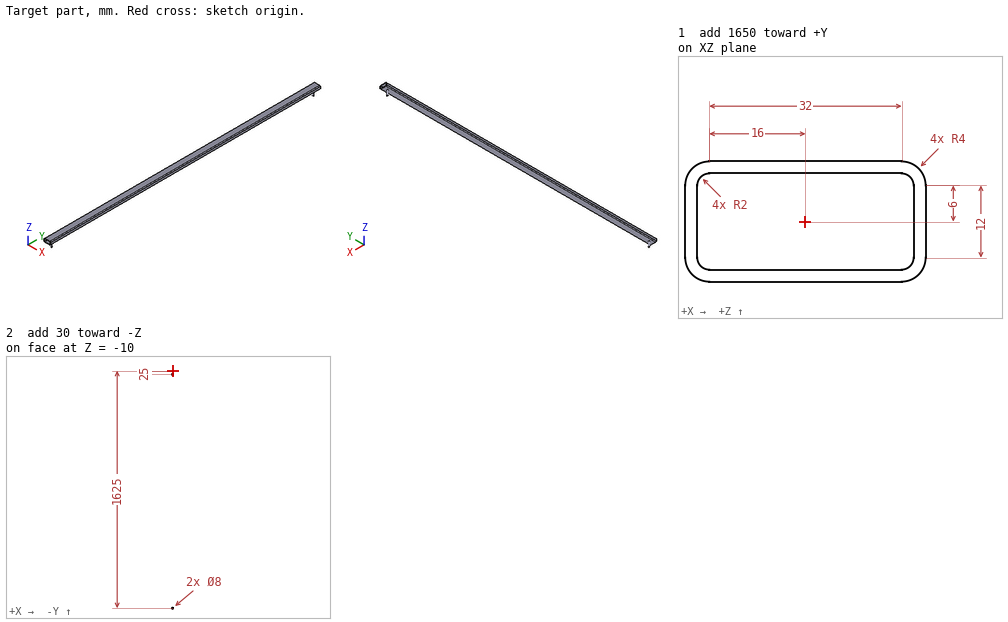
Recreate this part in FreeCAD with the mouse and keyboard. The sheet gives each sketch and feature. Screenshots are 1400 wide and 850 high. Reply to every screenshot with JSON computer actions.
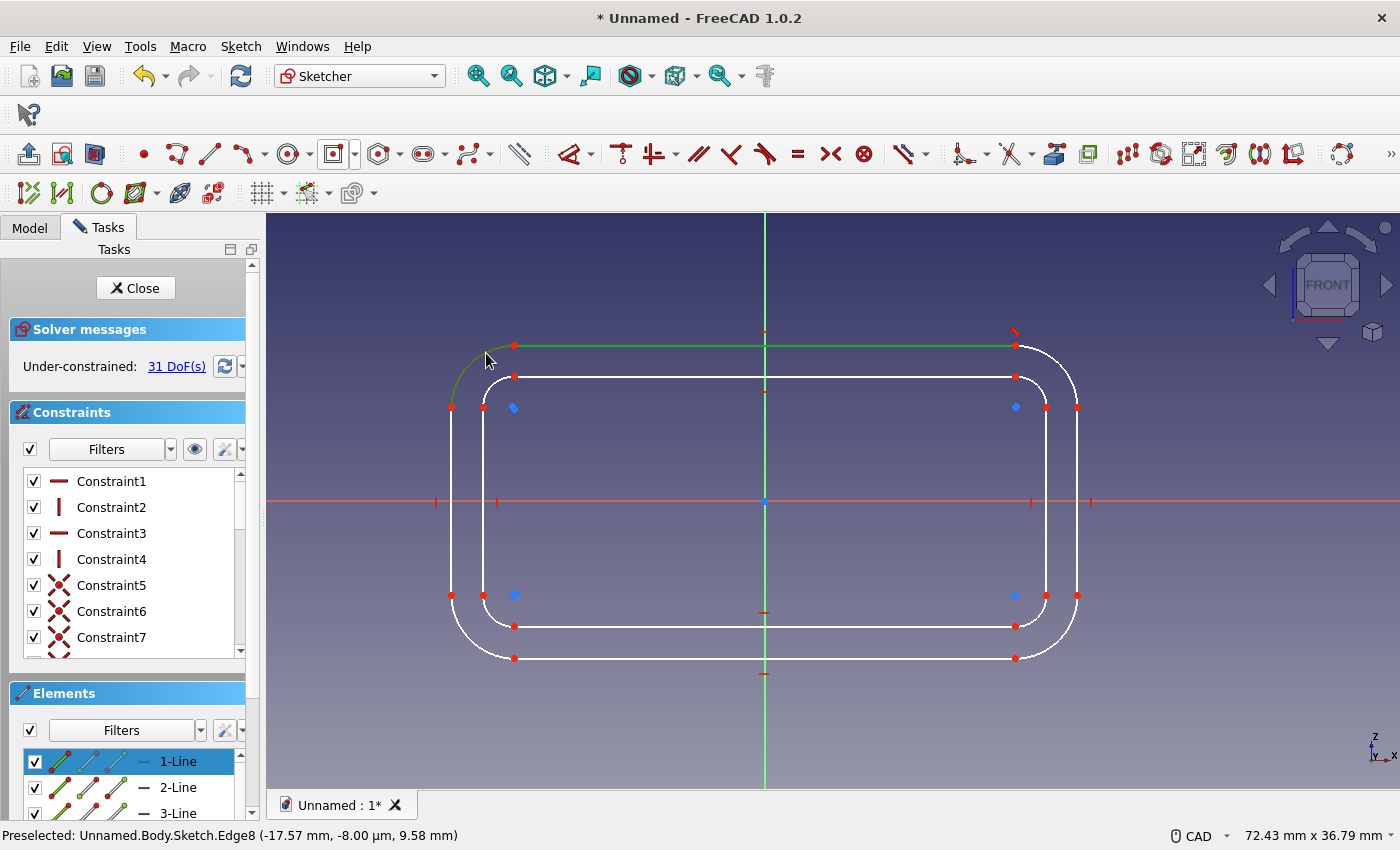
{"action": "key", "text": "t"}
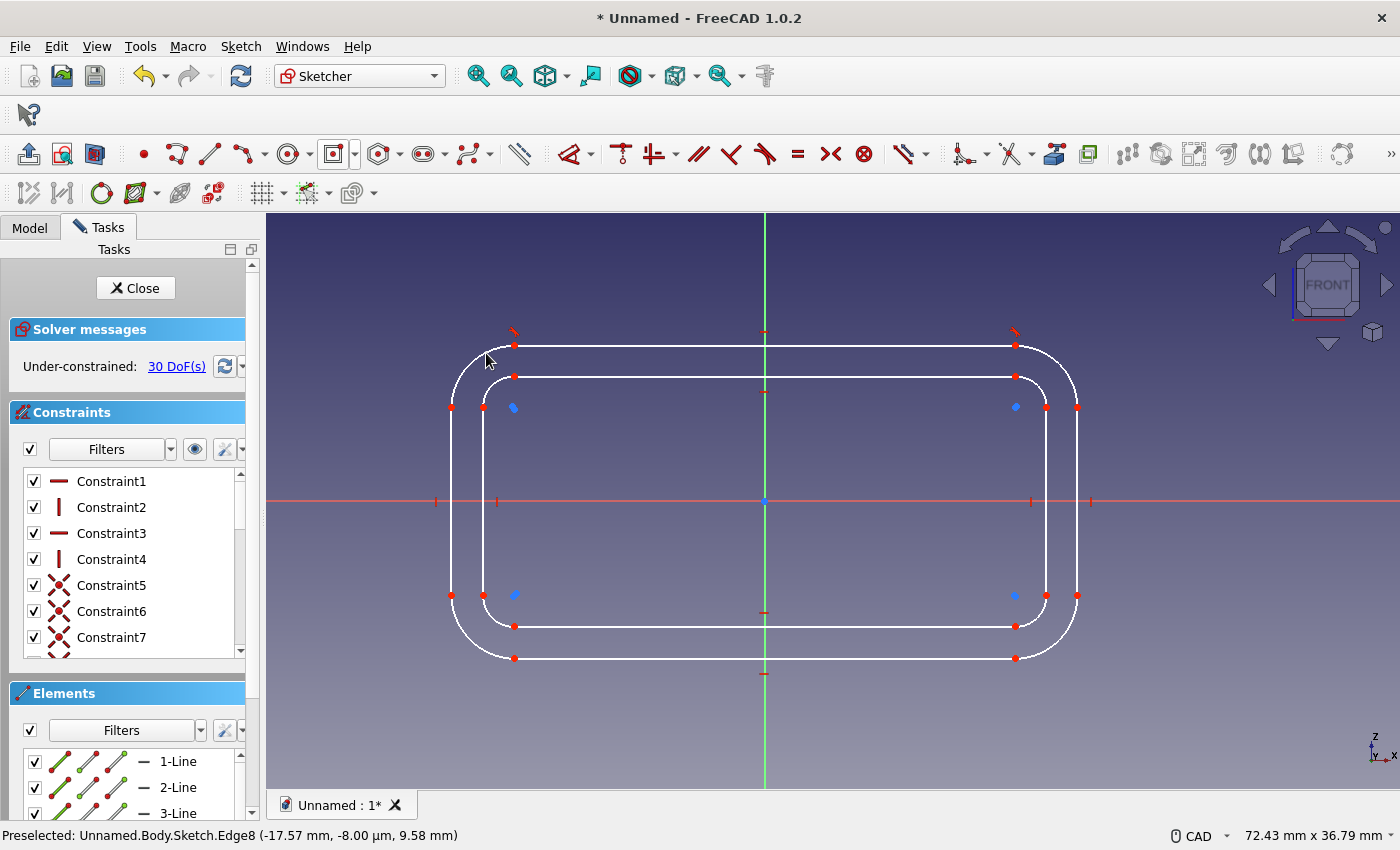
{"action": "left_click", "coordinate": [1077, 464]}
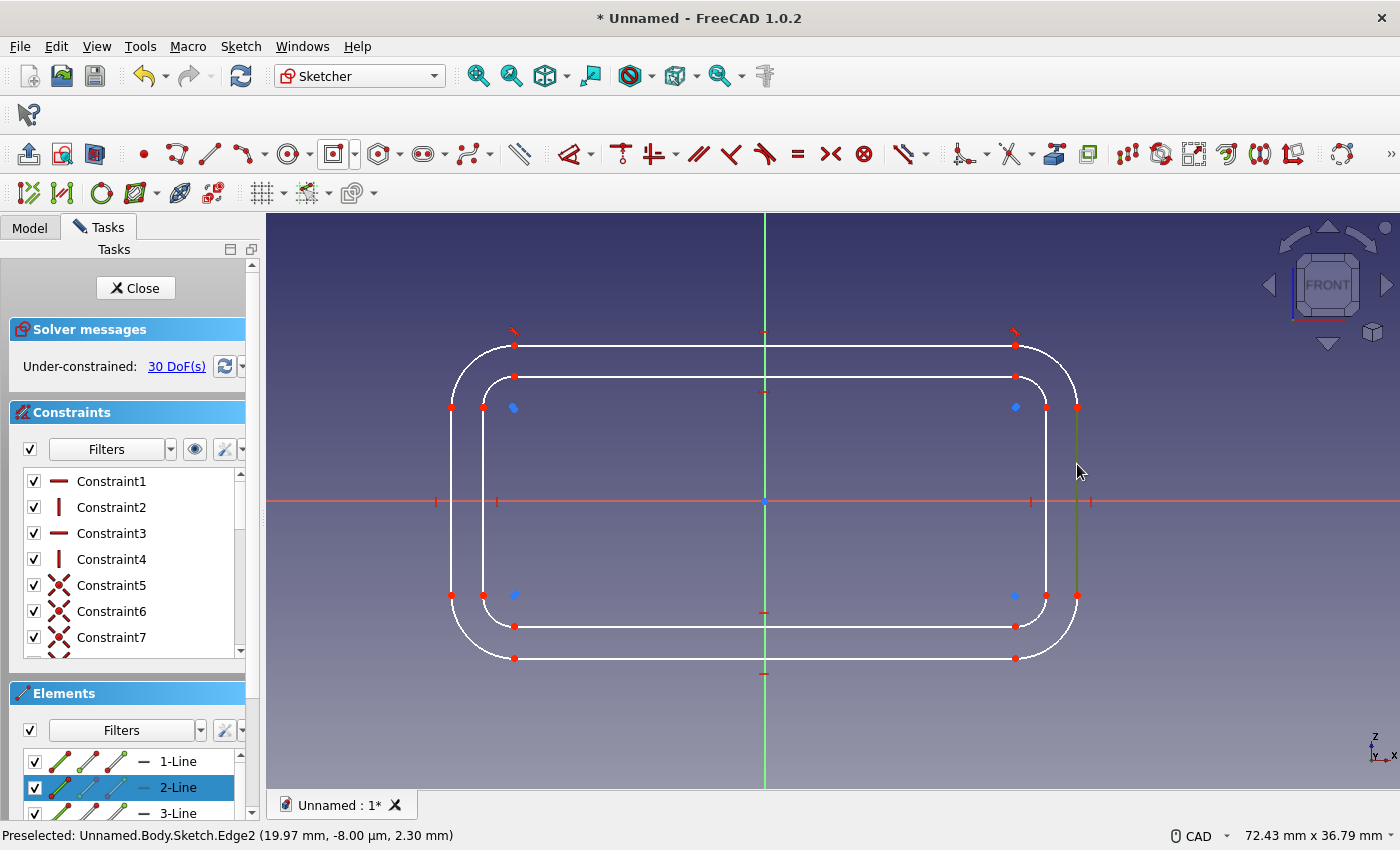
{"action": "left_click", "coordinate": [1071, 380]}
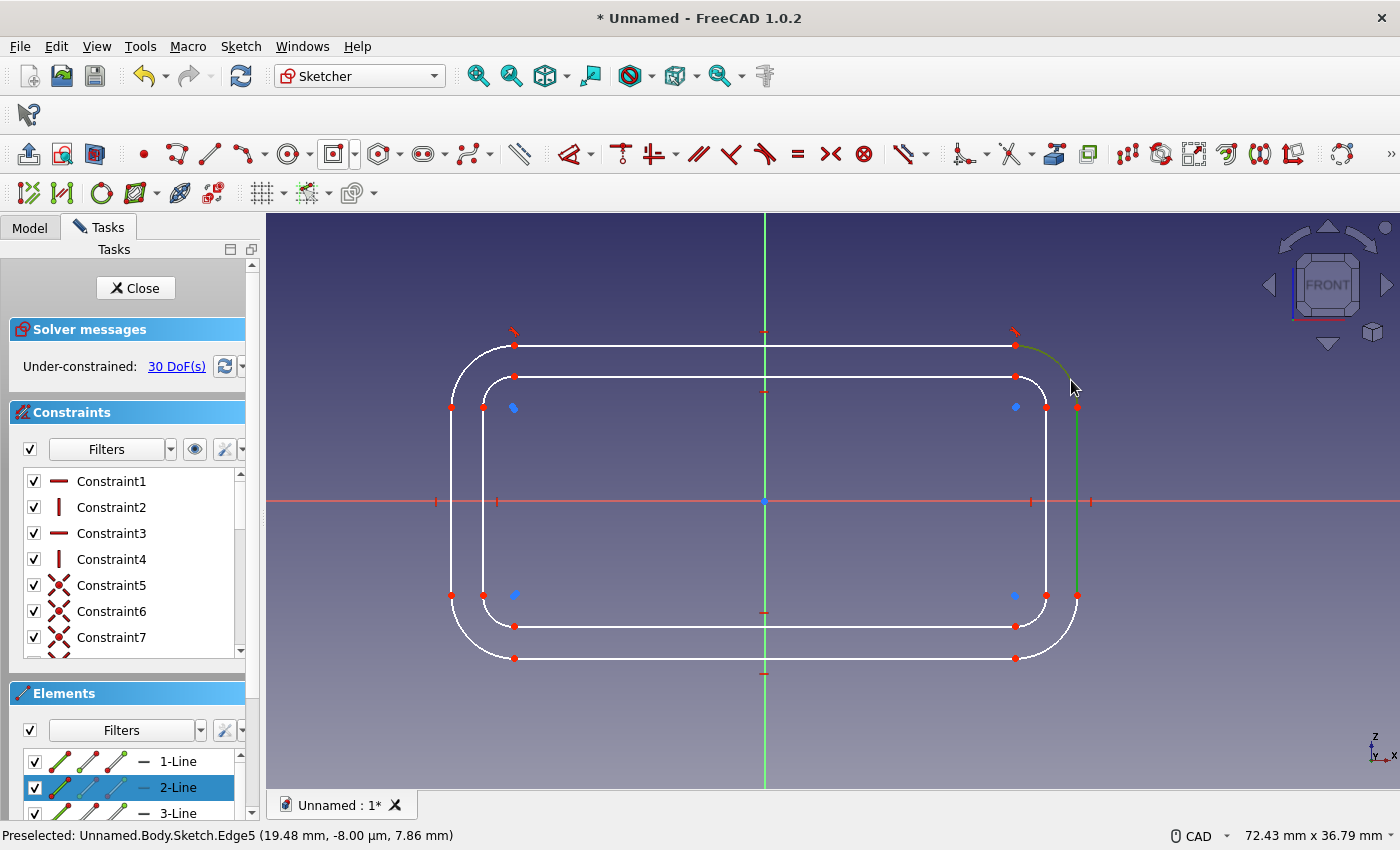
{"action": "left_click", "coordinate": [765, 154]}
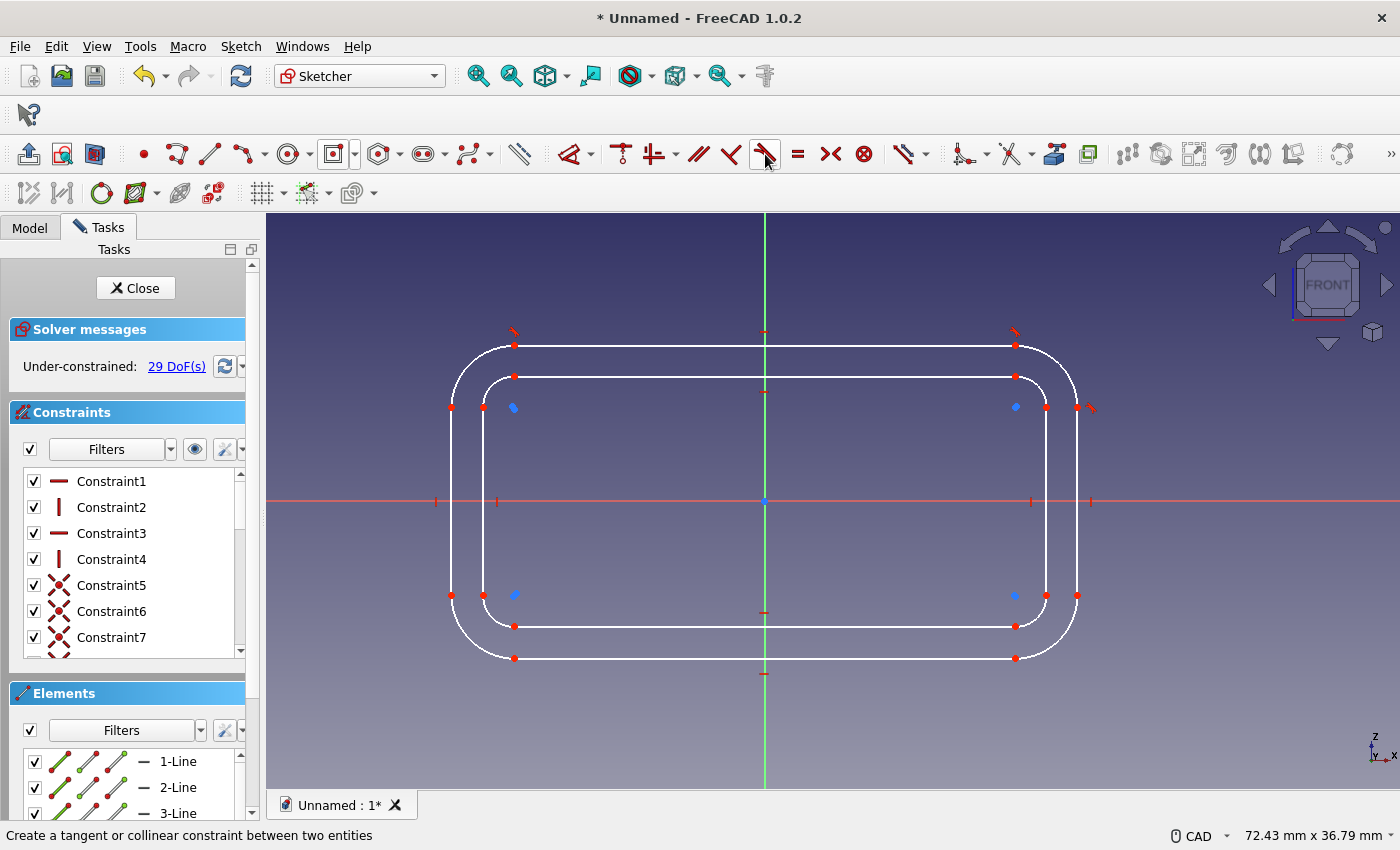
{"action": "left_click", "coordinate": [1077, 464]}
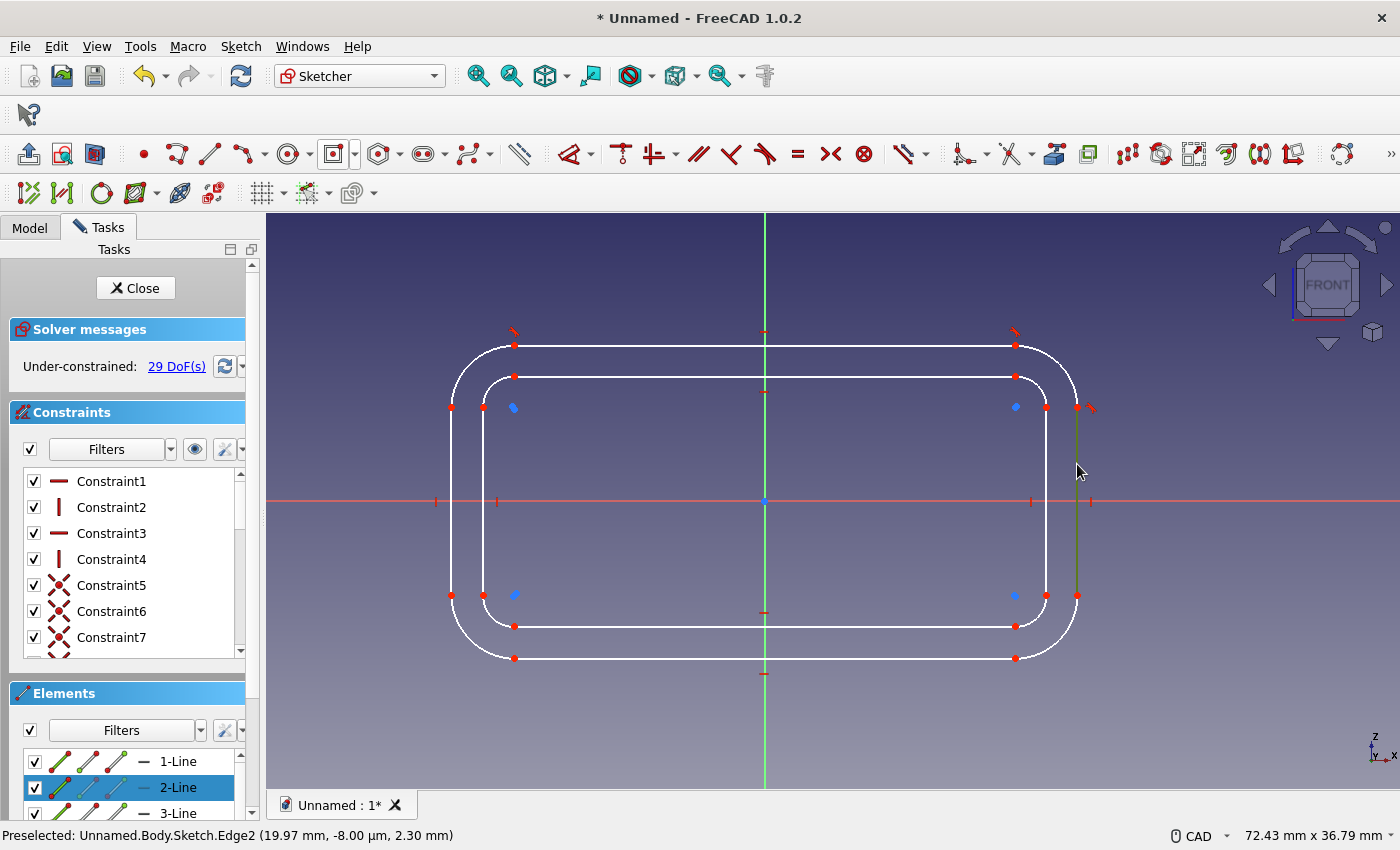
{"action": "left_click", "coordinate": [1044, 652]}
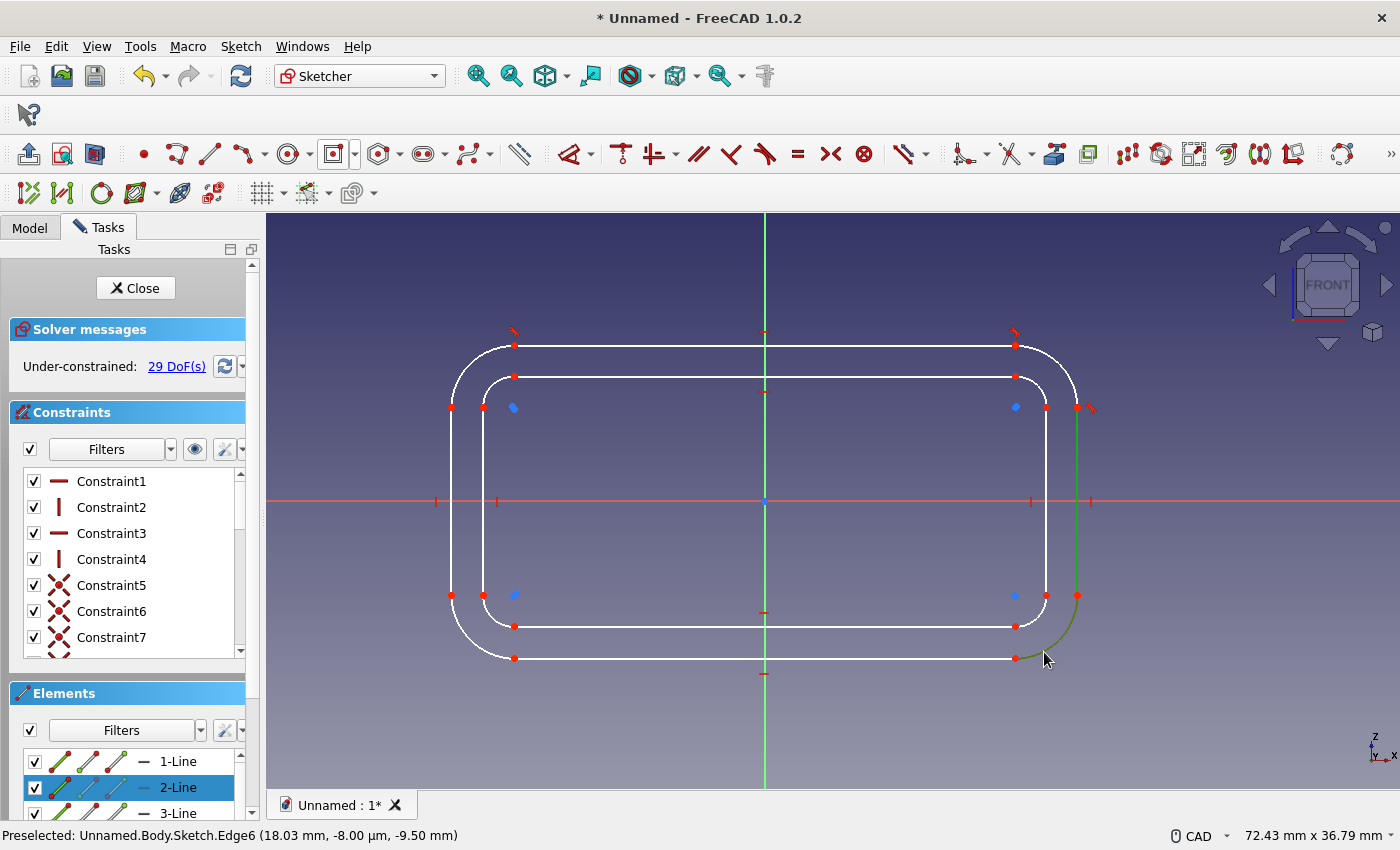
{"action": "left_click", "coordinate": [765, 154]}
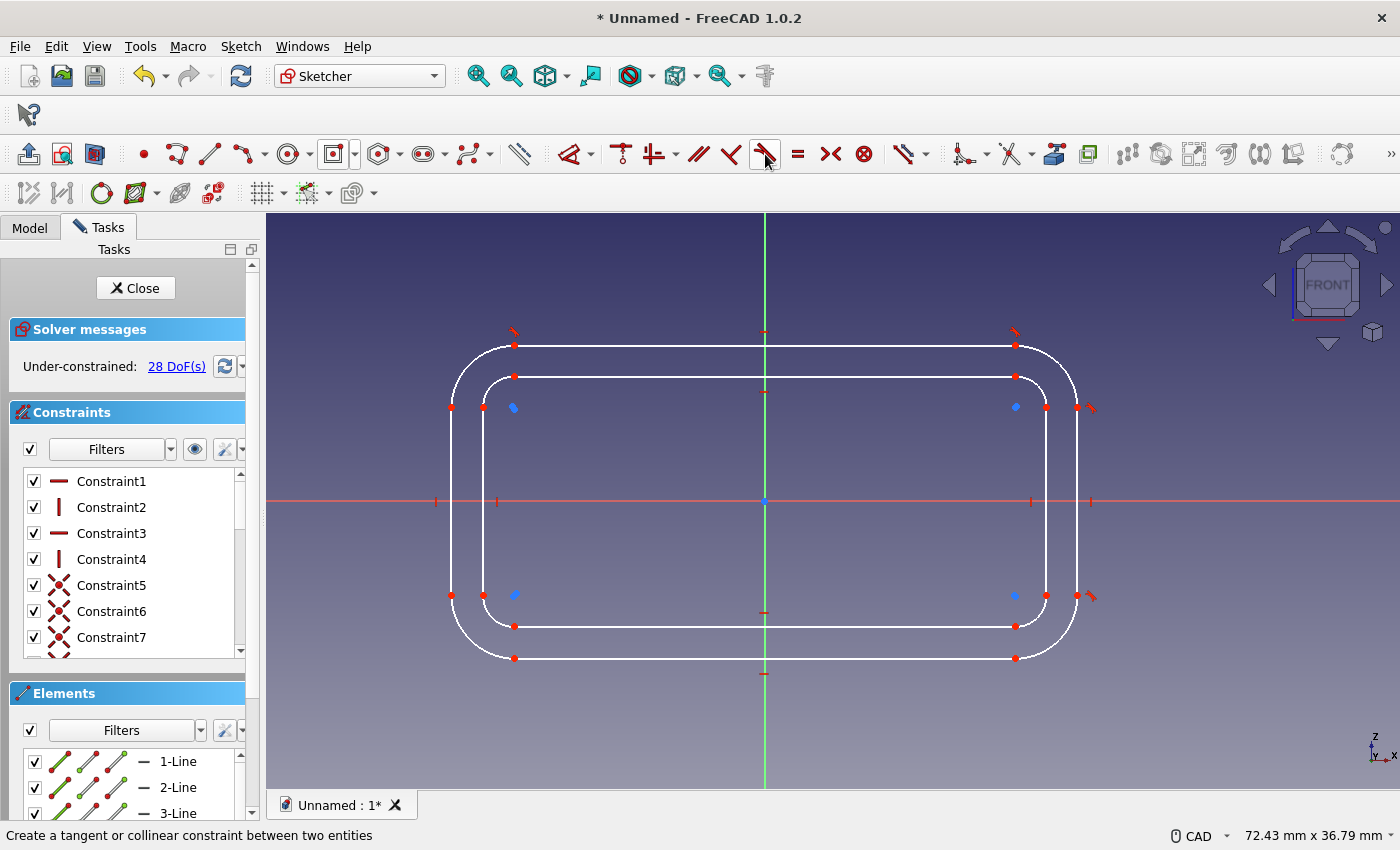
{"action": "left_click", "coordinate": [865, 659]}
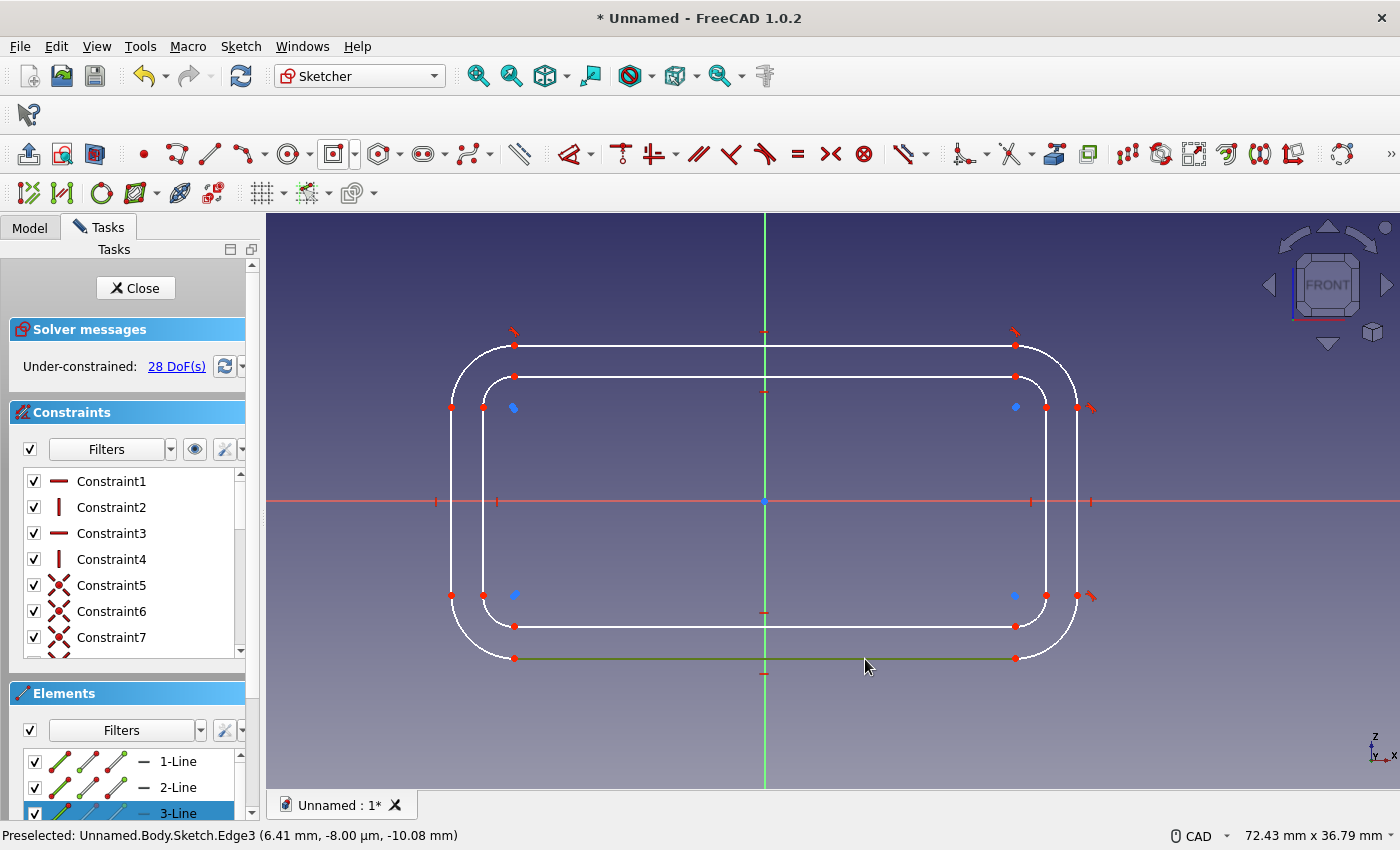
{"action": "left_click", "coordinate": [1044, 652]}